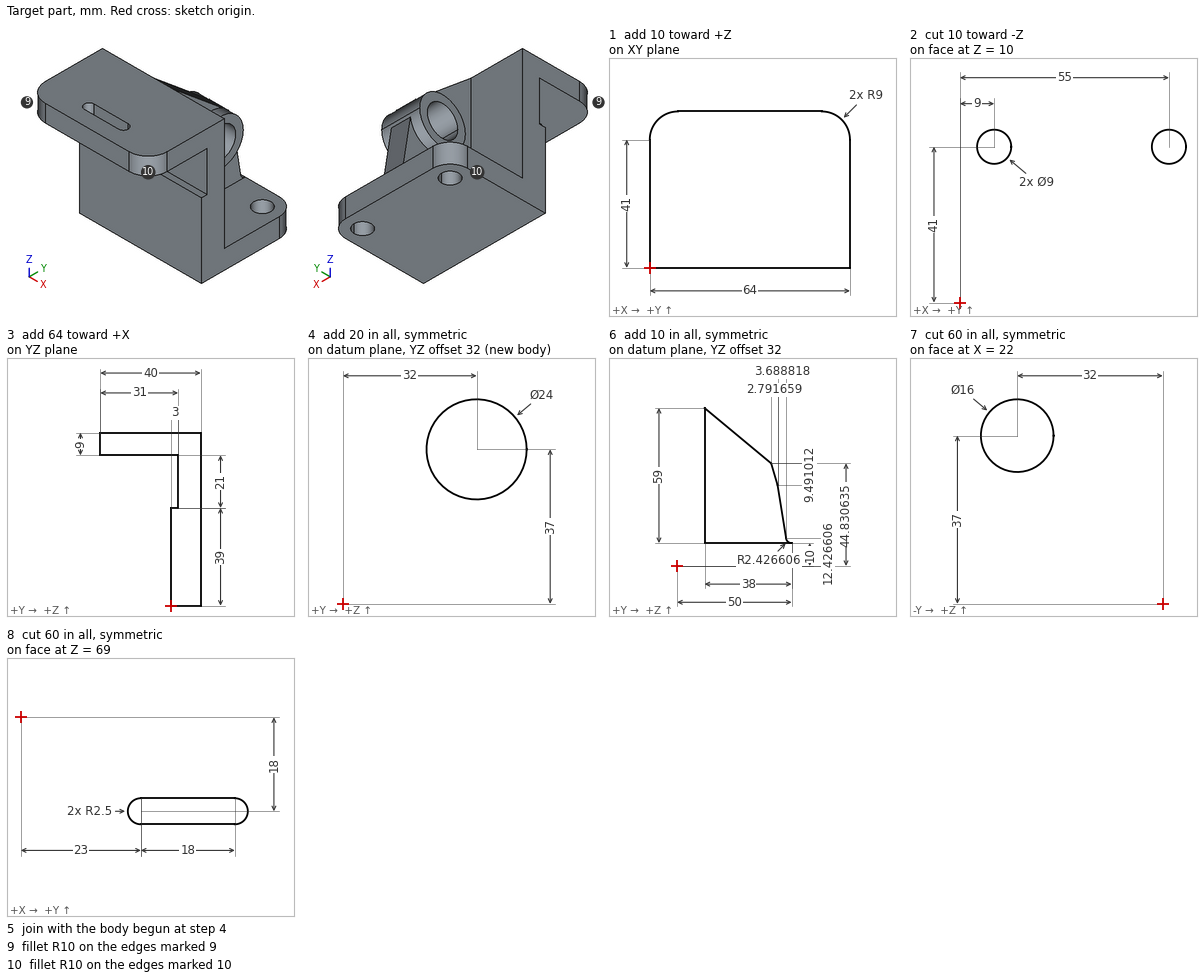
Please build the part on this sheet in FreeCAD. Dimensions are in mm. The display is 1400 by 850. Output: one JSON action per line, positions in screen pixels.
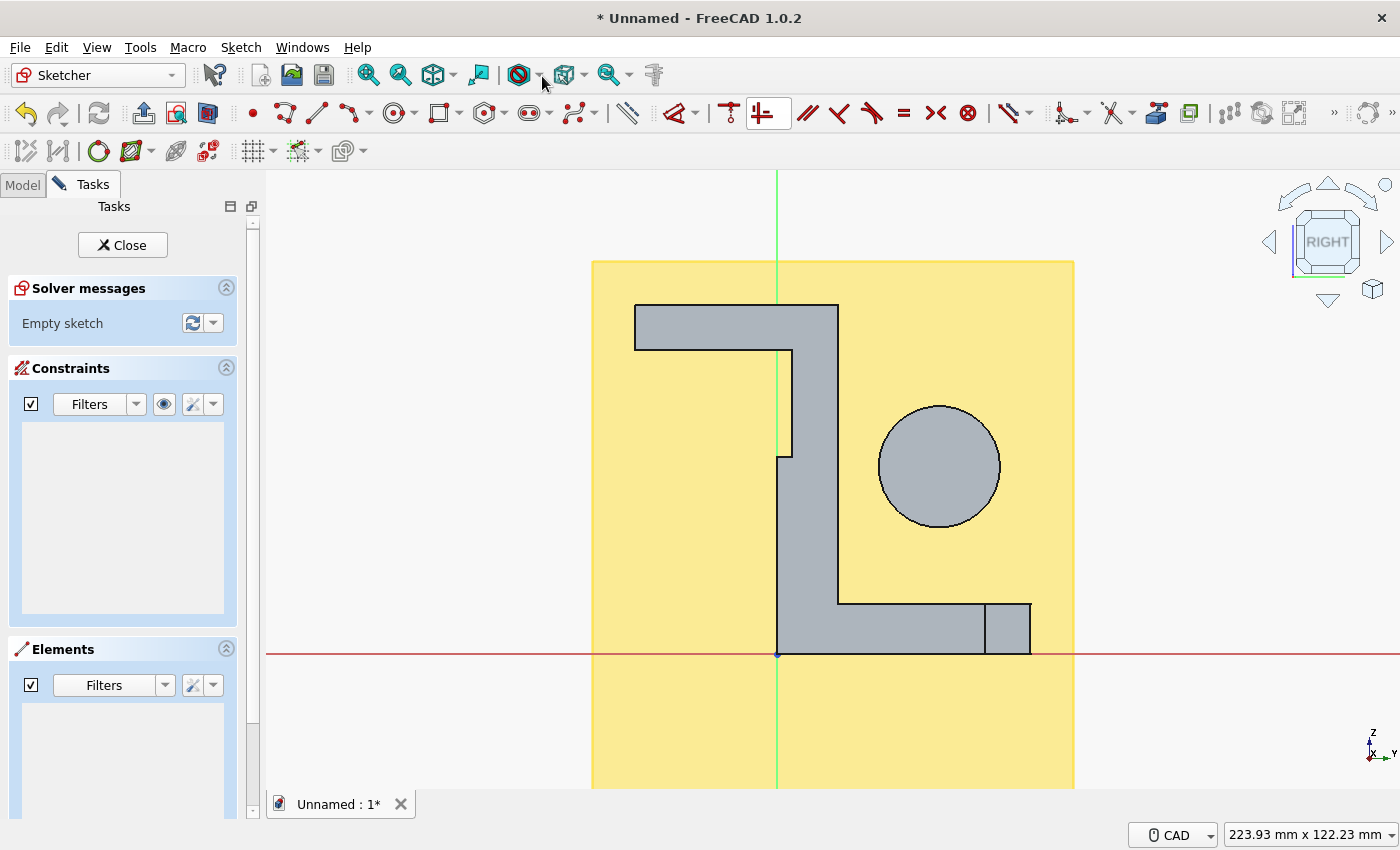
{"action": "left_click", "coordinate": [208, 114]}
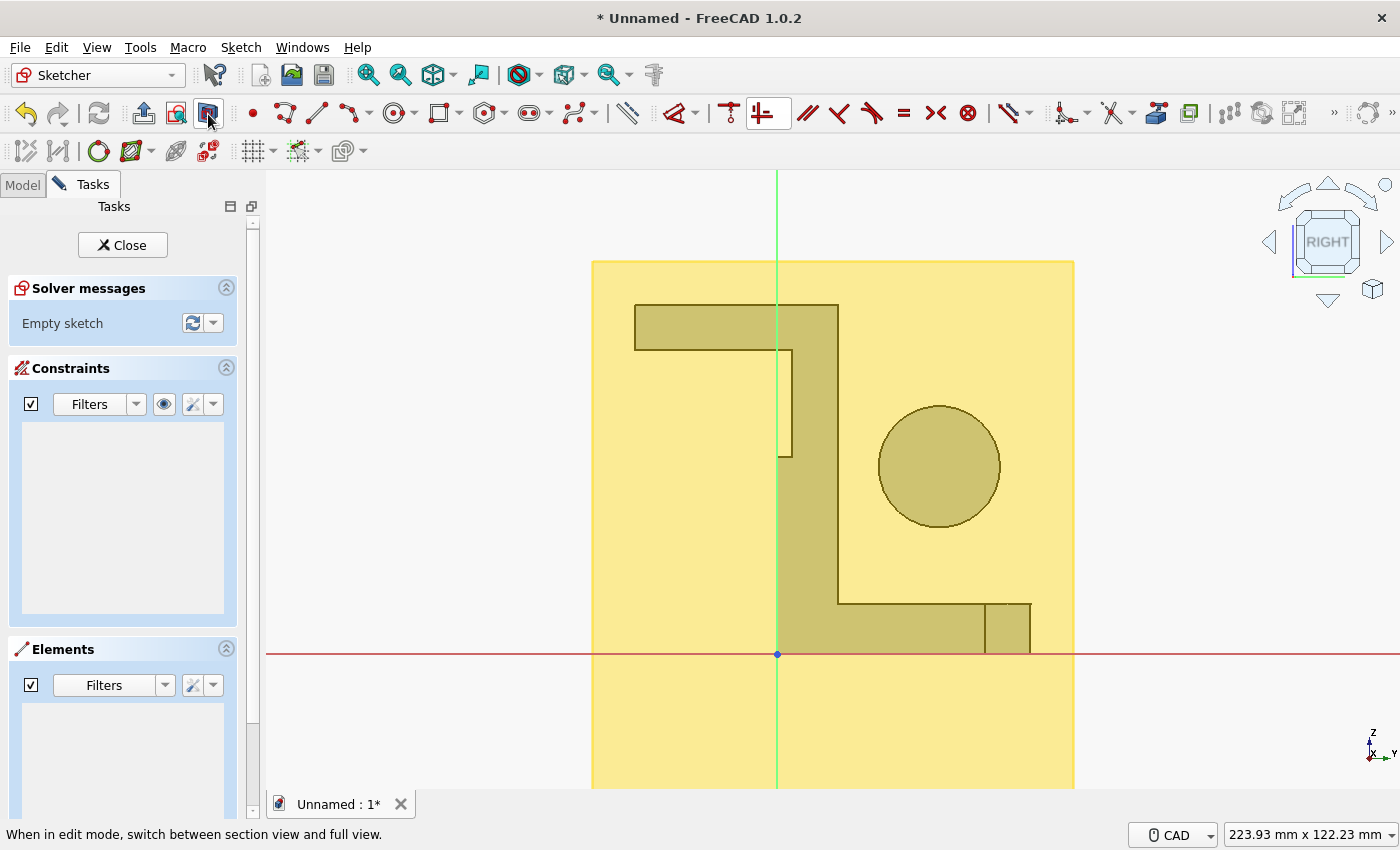
{"action": "left_click", "coordinate": [286, 114]}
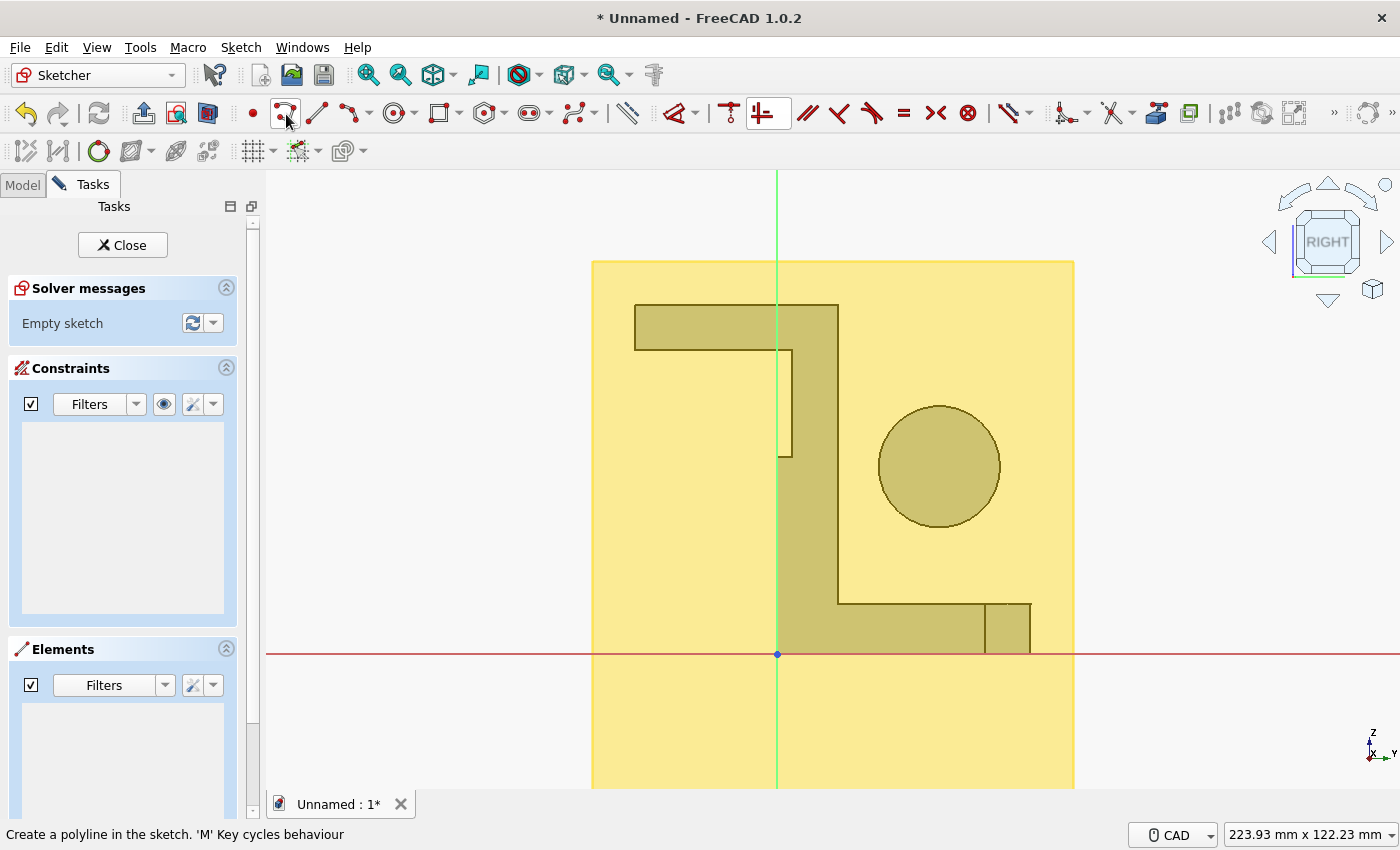
{"action": "left_click", "coordinate": [1030, 604]}
{"action": "left_click", "coordinate": [838, 604]}
{"action": "left_click", "coordinate": [838, 305]}
{"action": "left_click", "coordinate": [985, 427]}
{"action": "left_click", "coordinate": [1000, 475]}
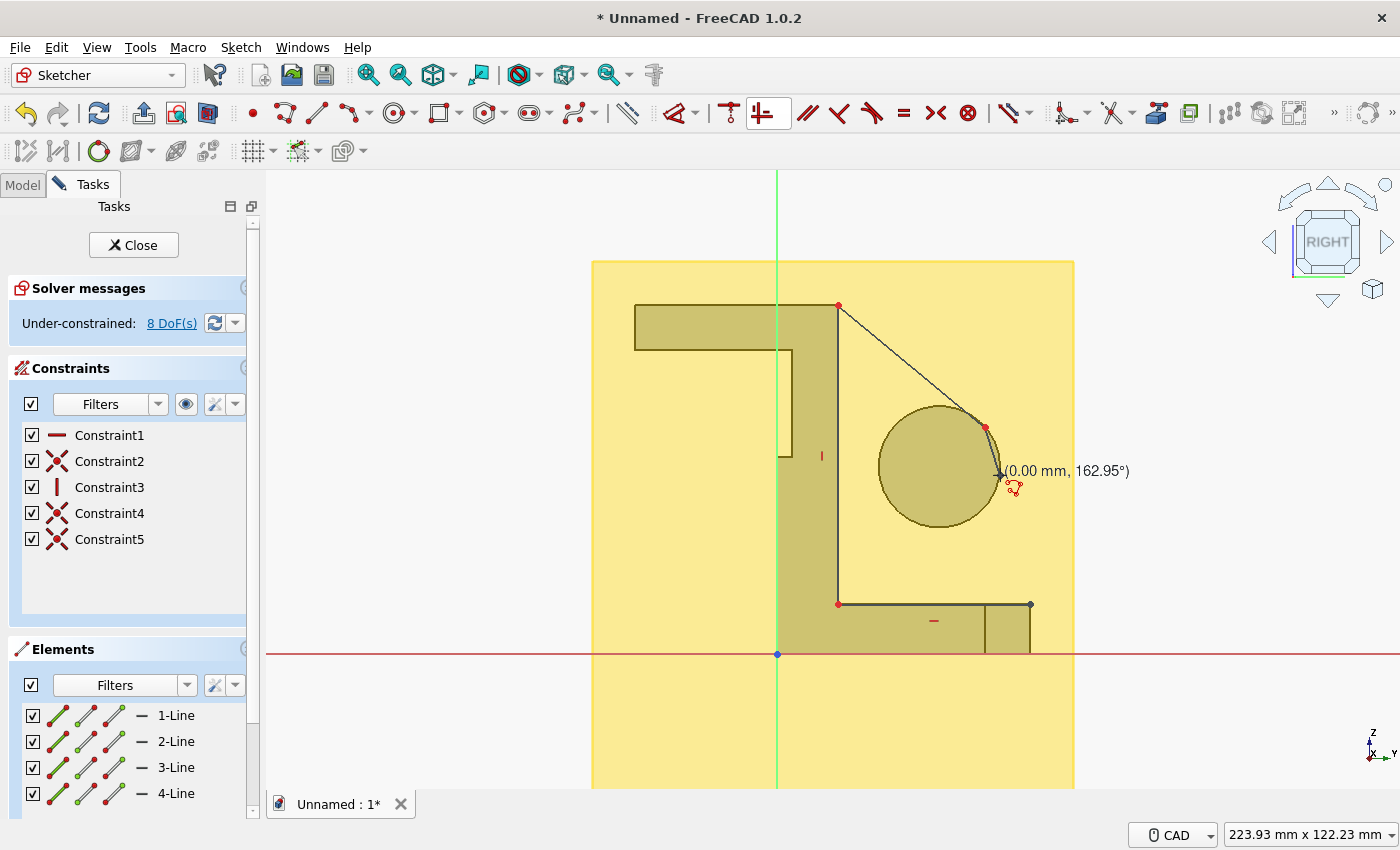
{"action": "scroll", "coordinate": [1018, 591], "scroll_direction": "up", "scroll_amount": 2}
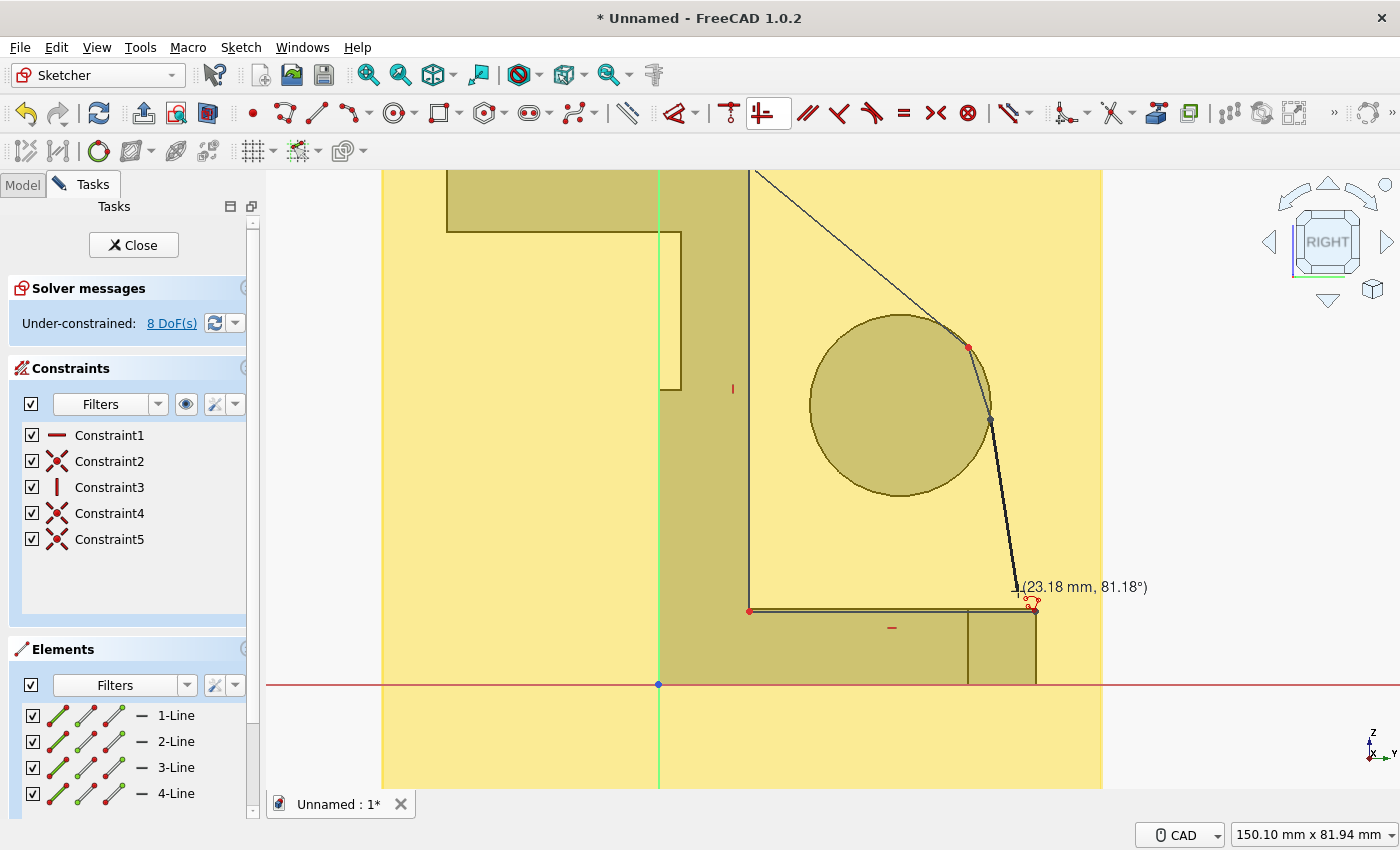
{"action": "left_click", "coordinate": [1018, 591]}
{"action": "right_click", "coordinate": [1018, 591]}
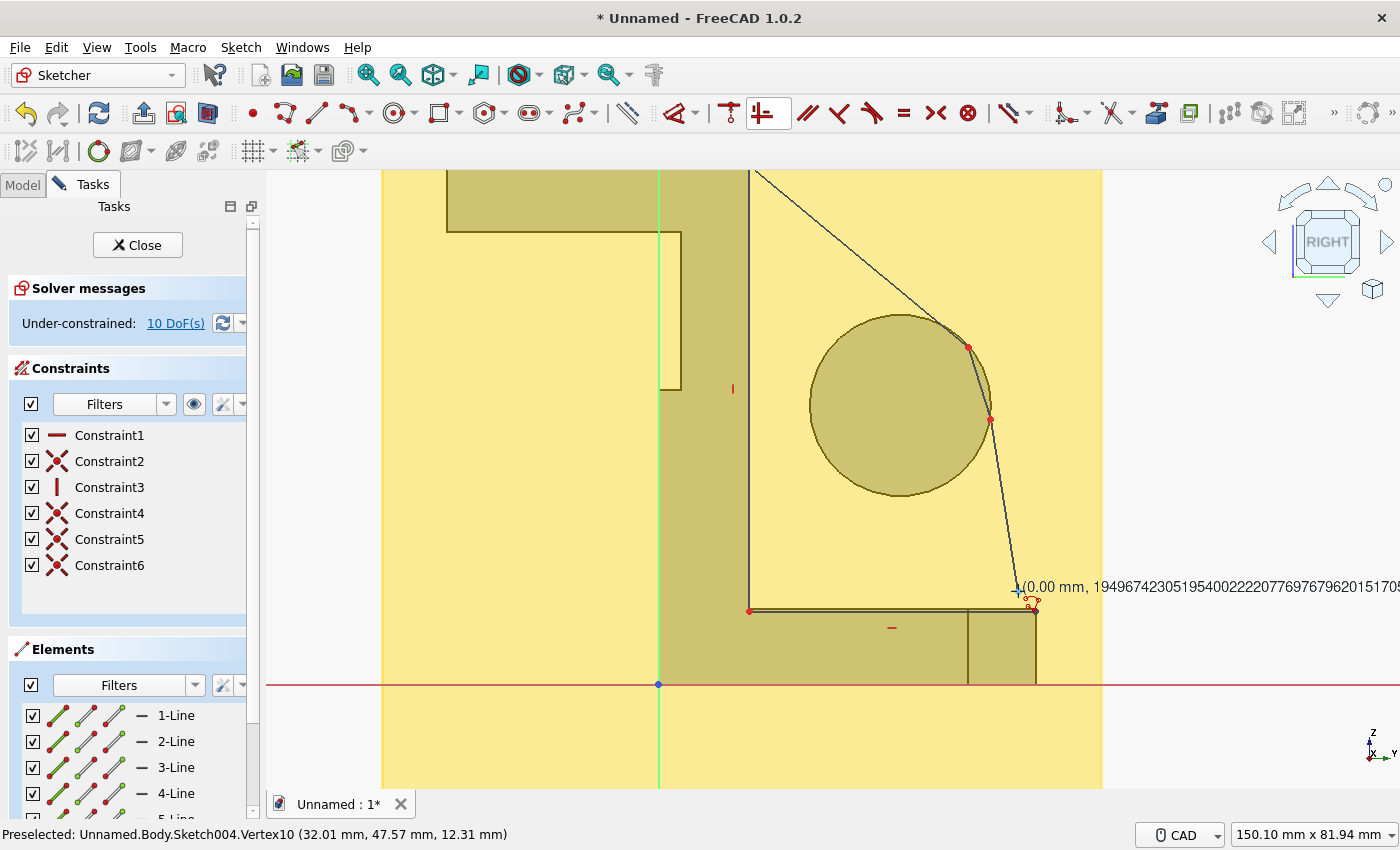
{"action": "left_click", "coordinate": [350, 114]}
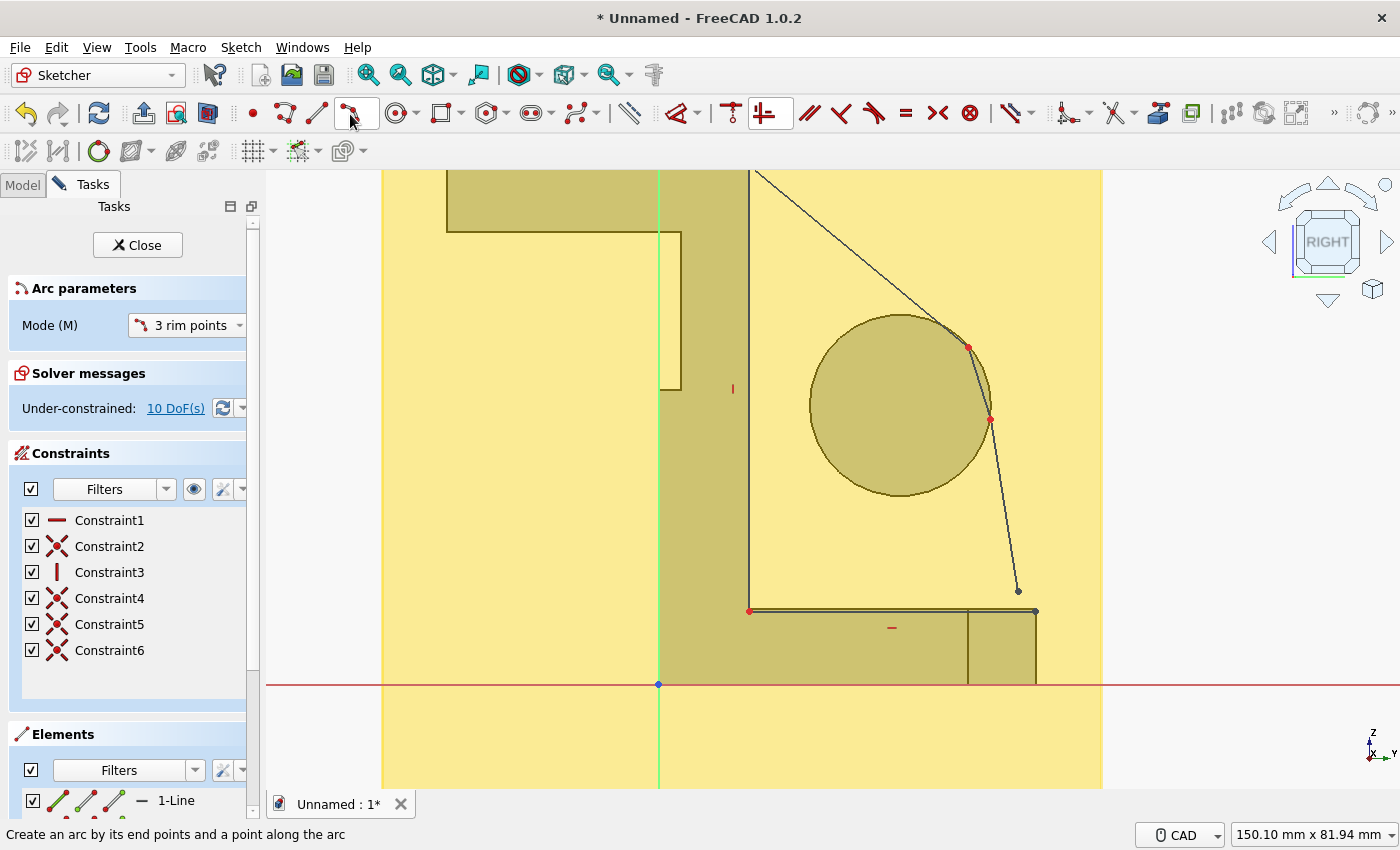
{"action": "left_click", "coordinate": [1018, 592]}
{"action": "left_click", "coordinate": [1036, 612]}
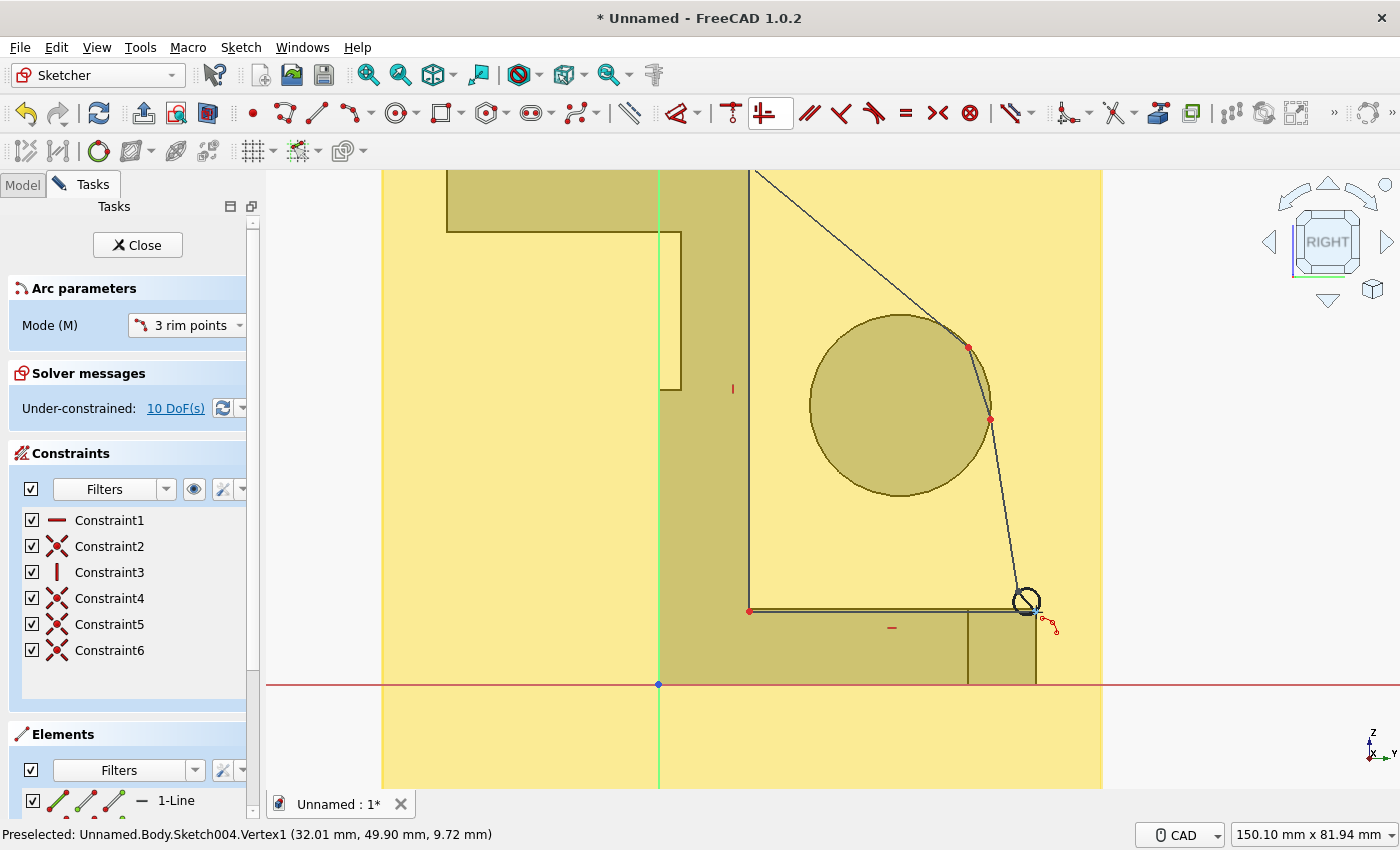
{"action": "scroll", "coordinate": [1023, 604], "scroll_direction": "up", "scroll_amount": 6}